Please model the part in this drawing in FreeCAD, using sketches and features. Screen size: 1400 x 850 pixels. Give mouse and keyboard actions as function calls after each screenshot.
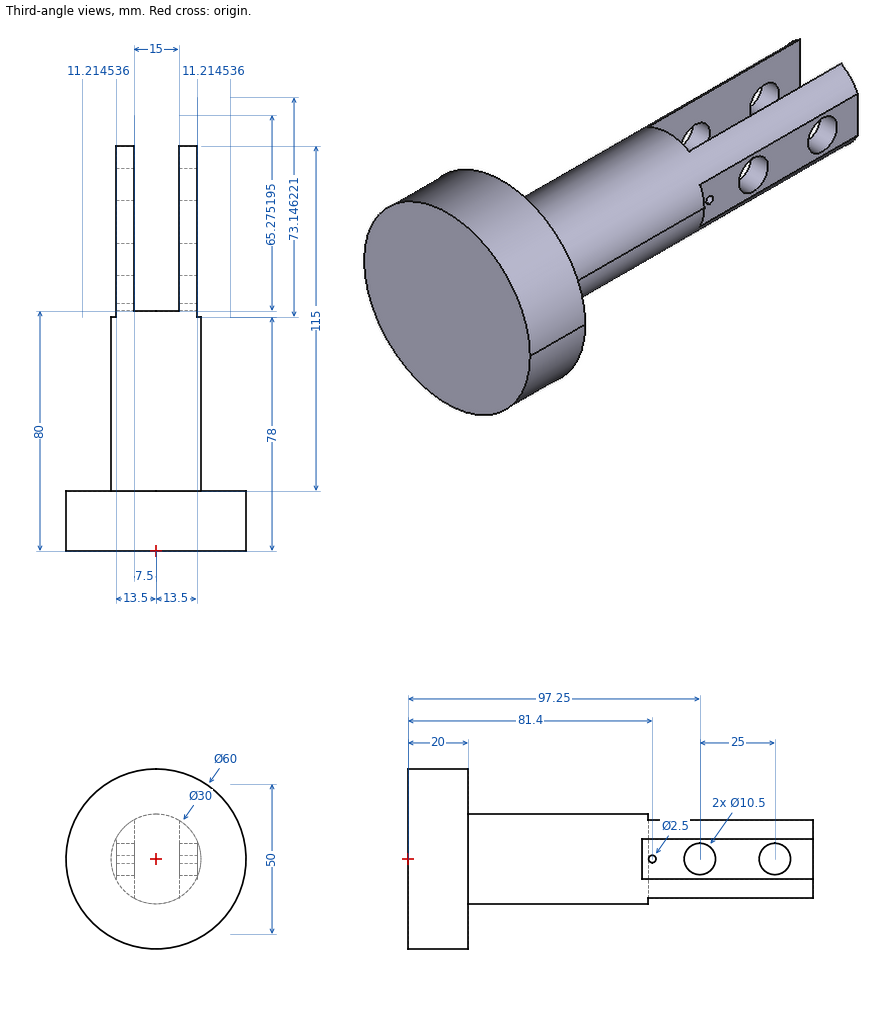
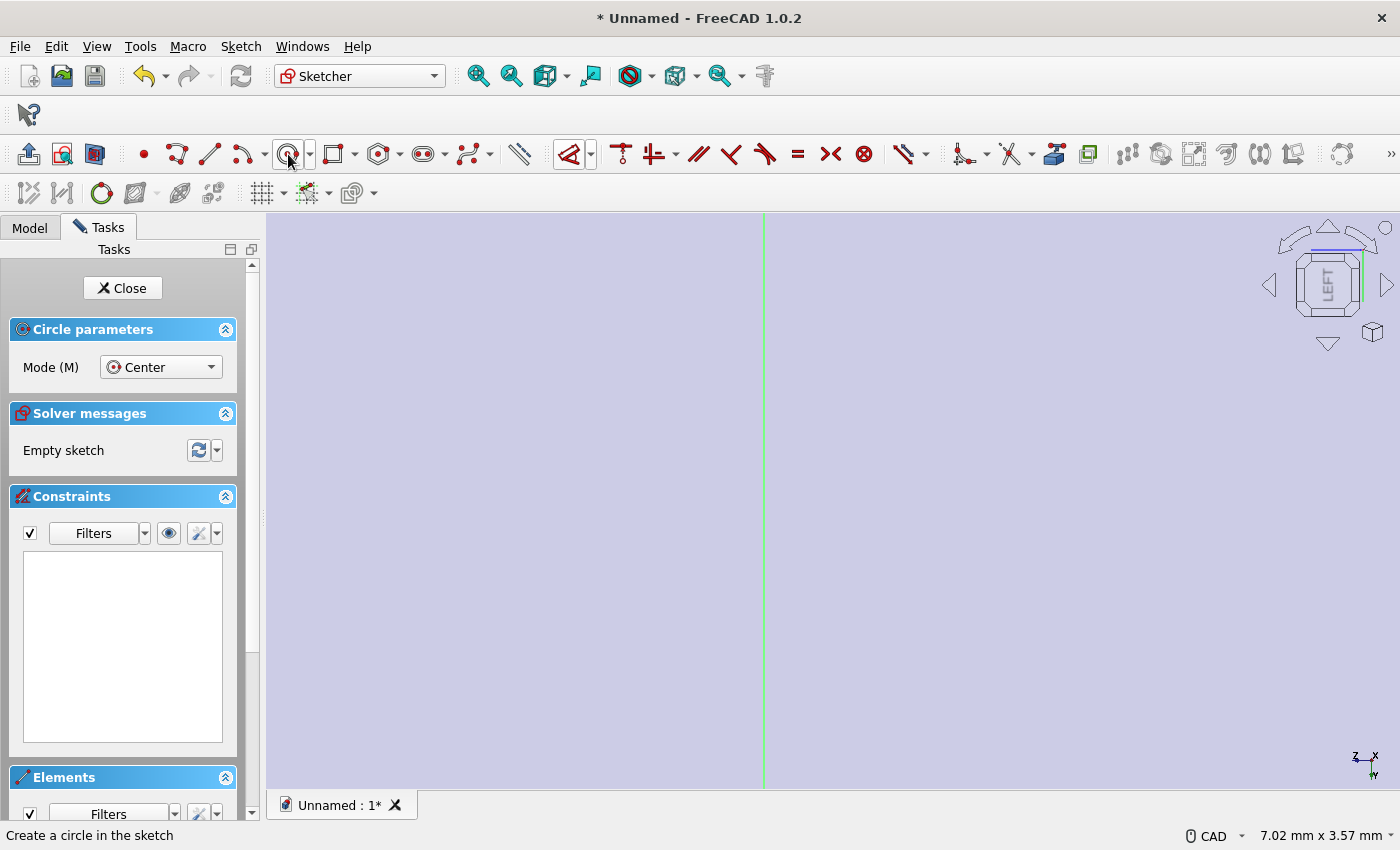
click(764, 500)
move(907, 357)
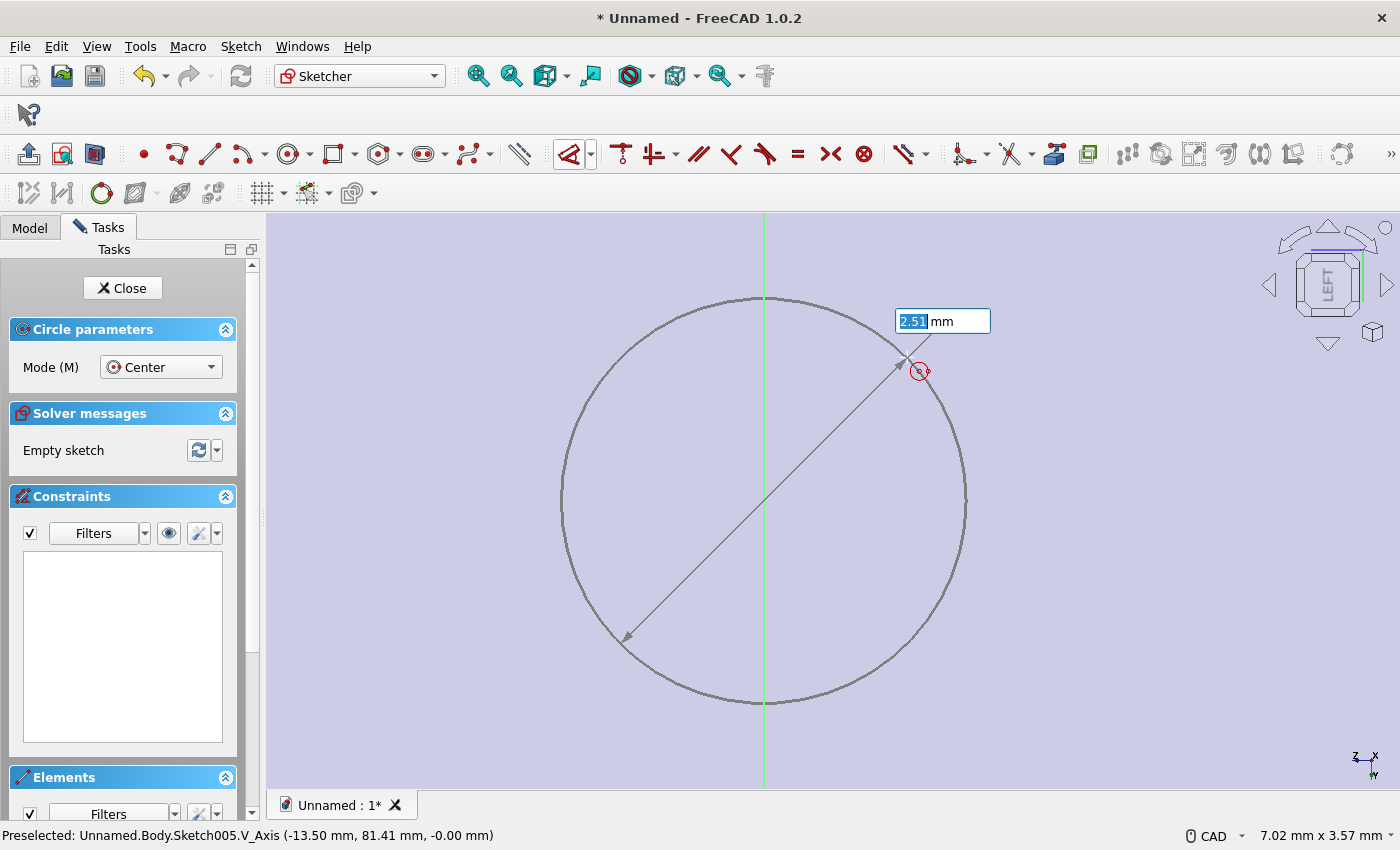
text(2.5)
key(Return)
key(Escape)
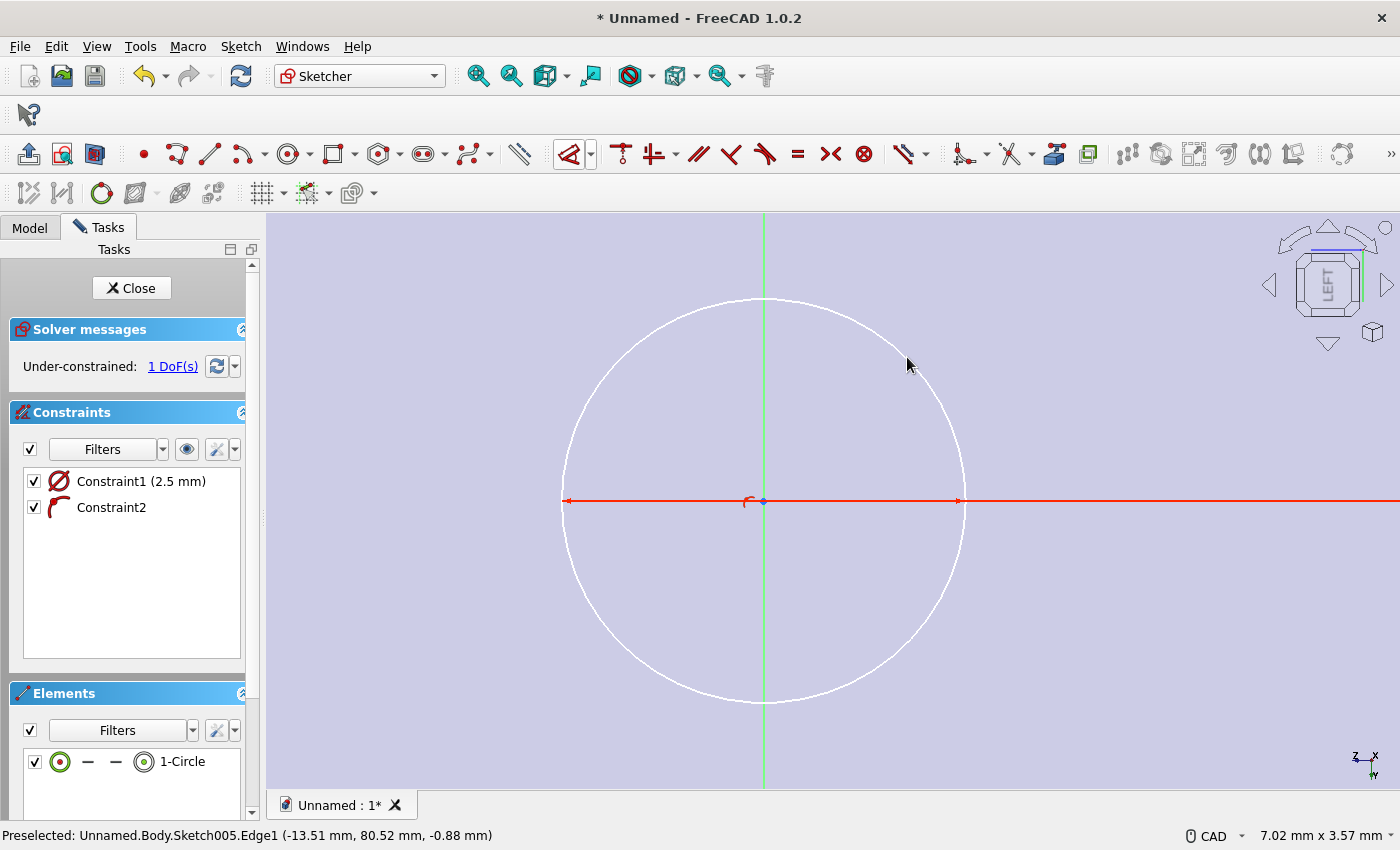
click(764, 501)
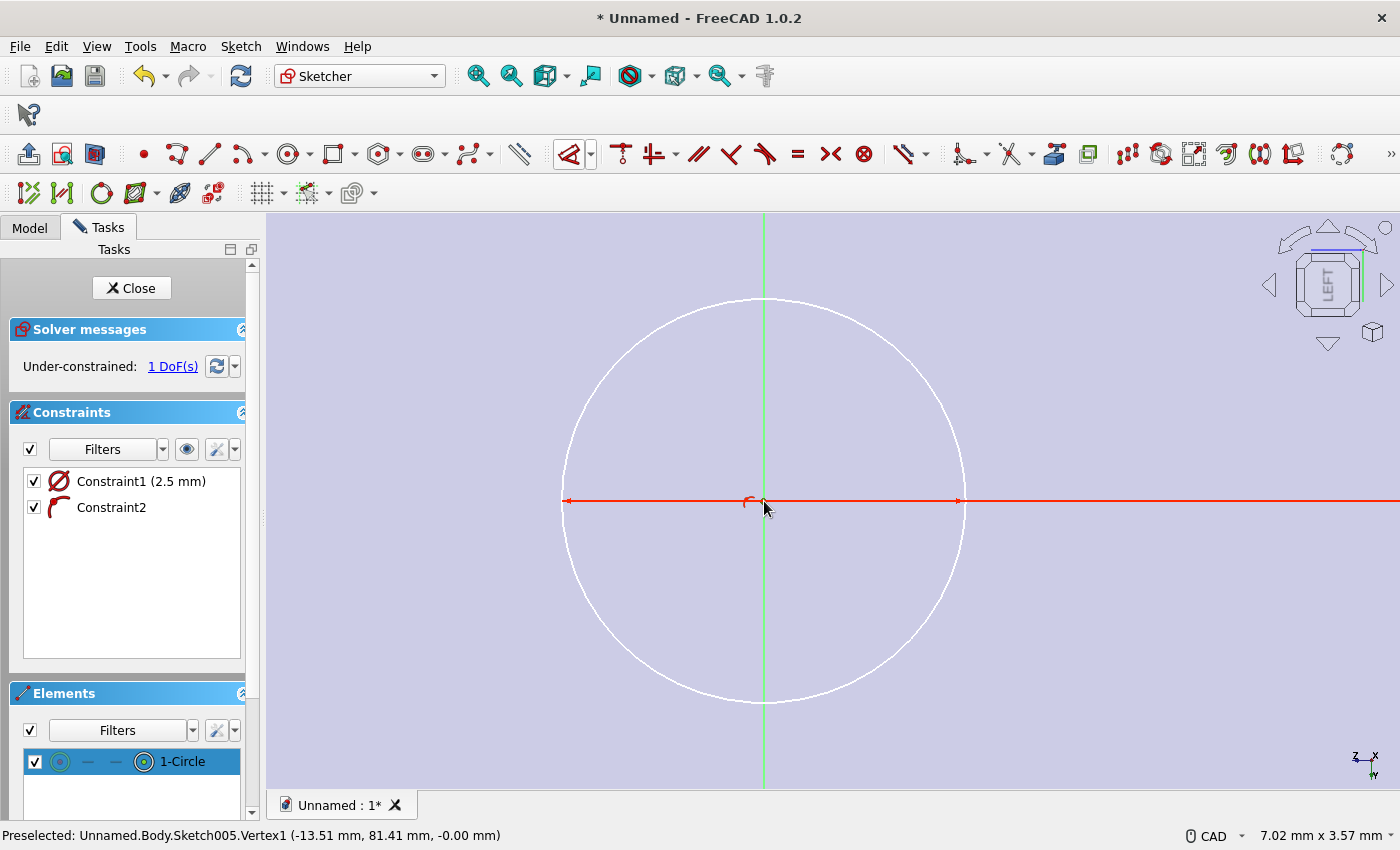
key(i)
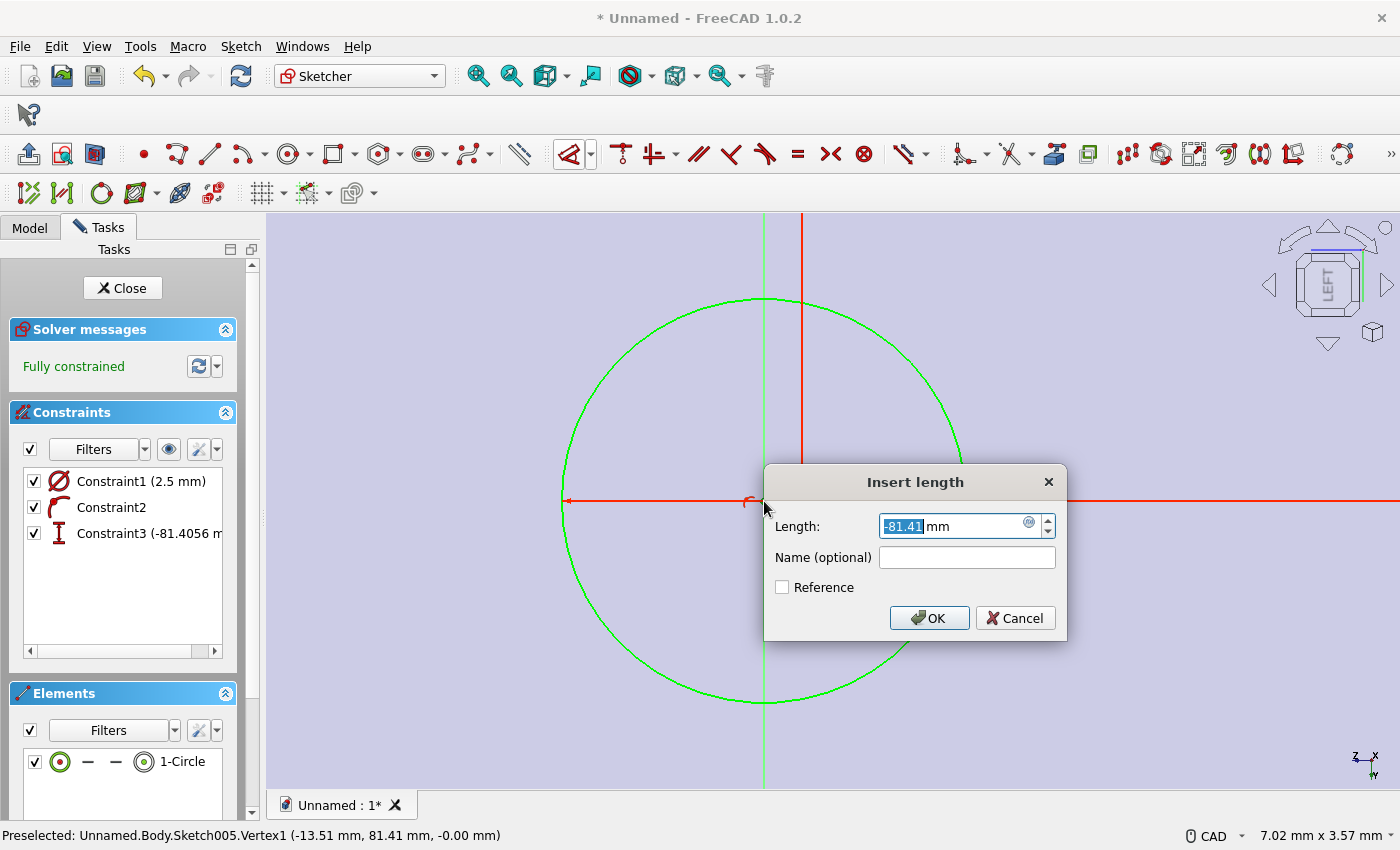
text(-81.4)
key(Return)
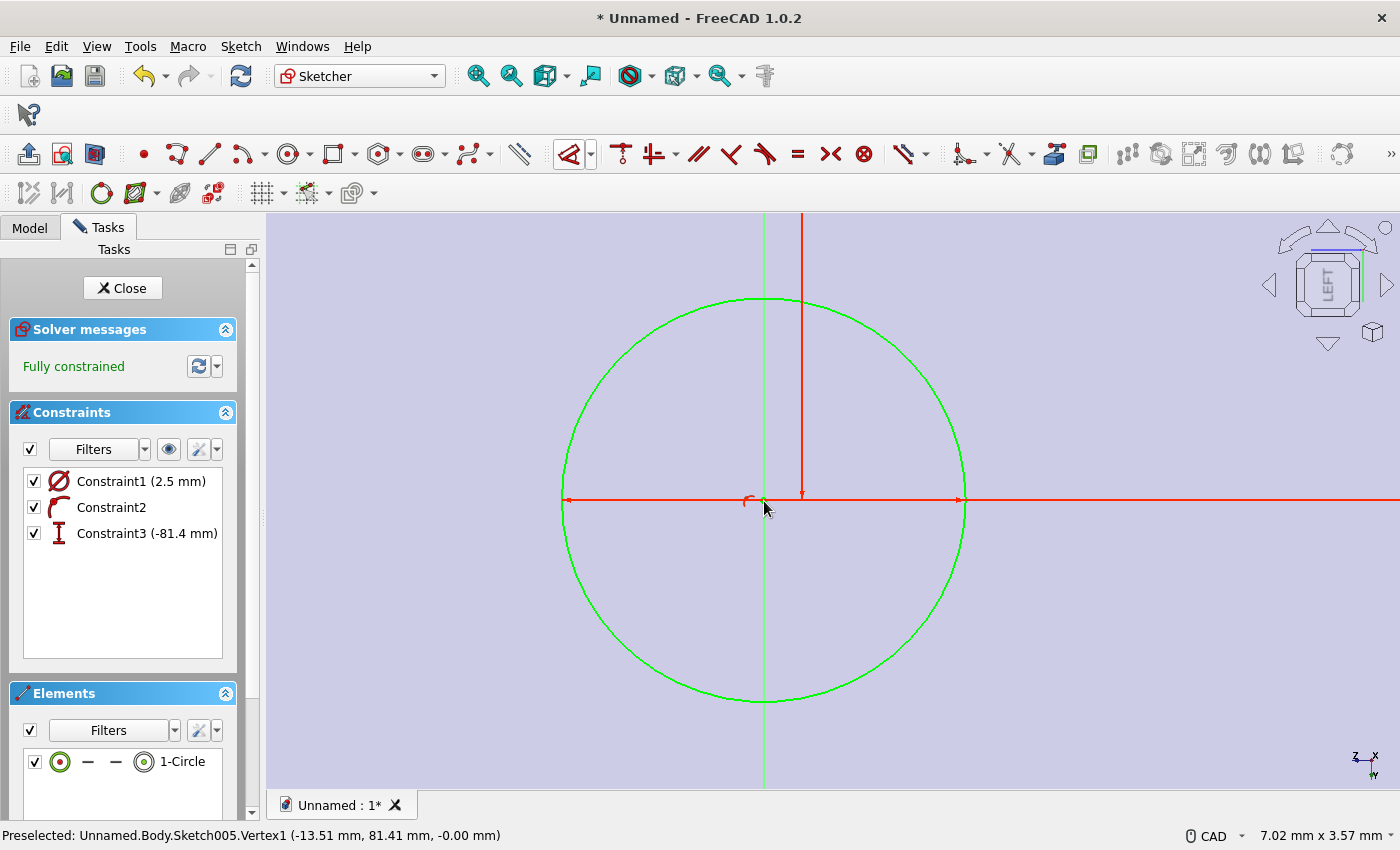
click(123, 288)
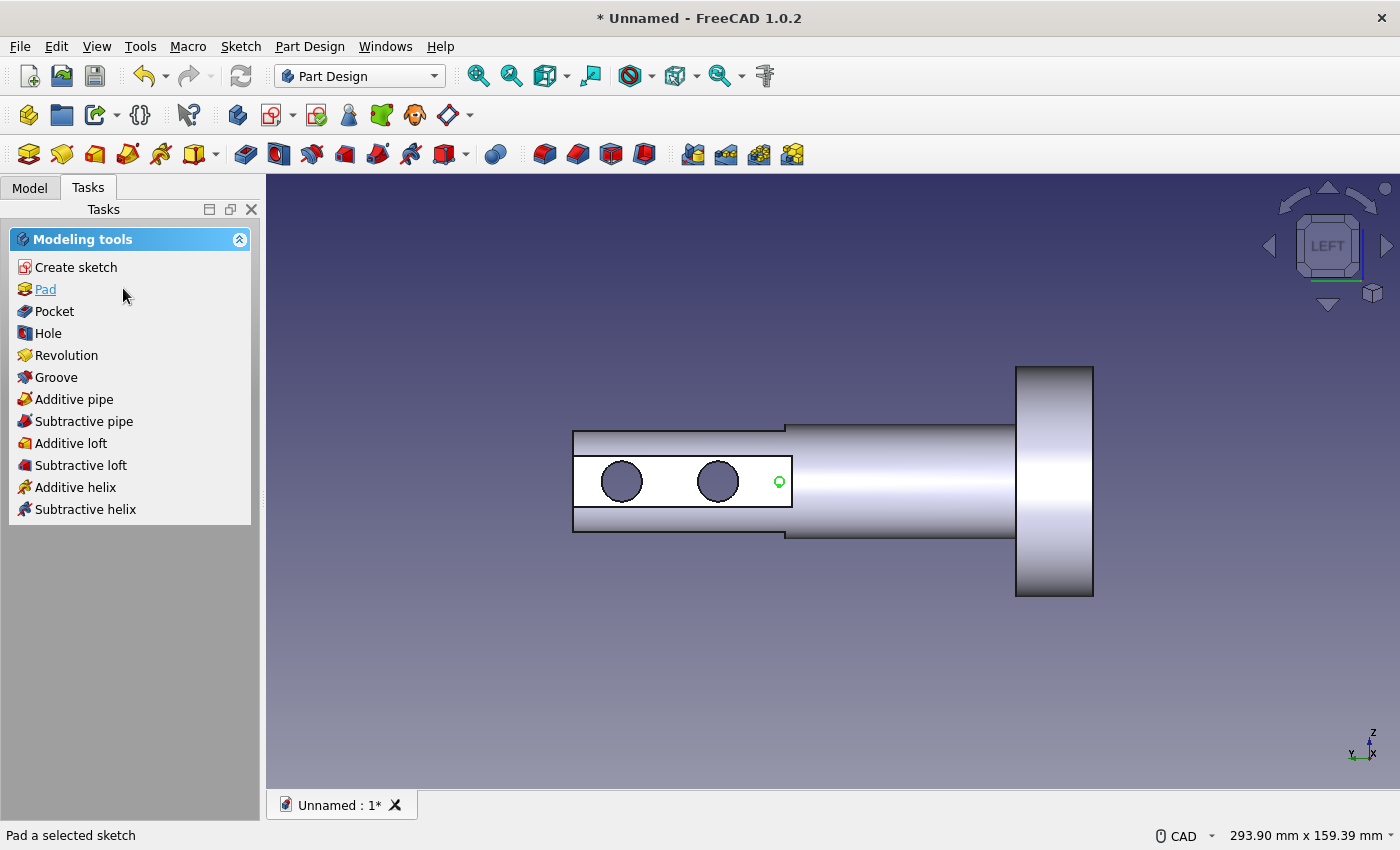
click(246, 154)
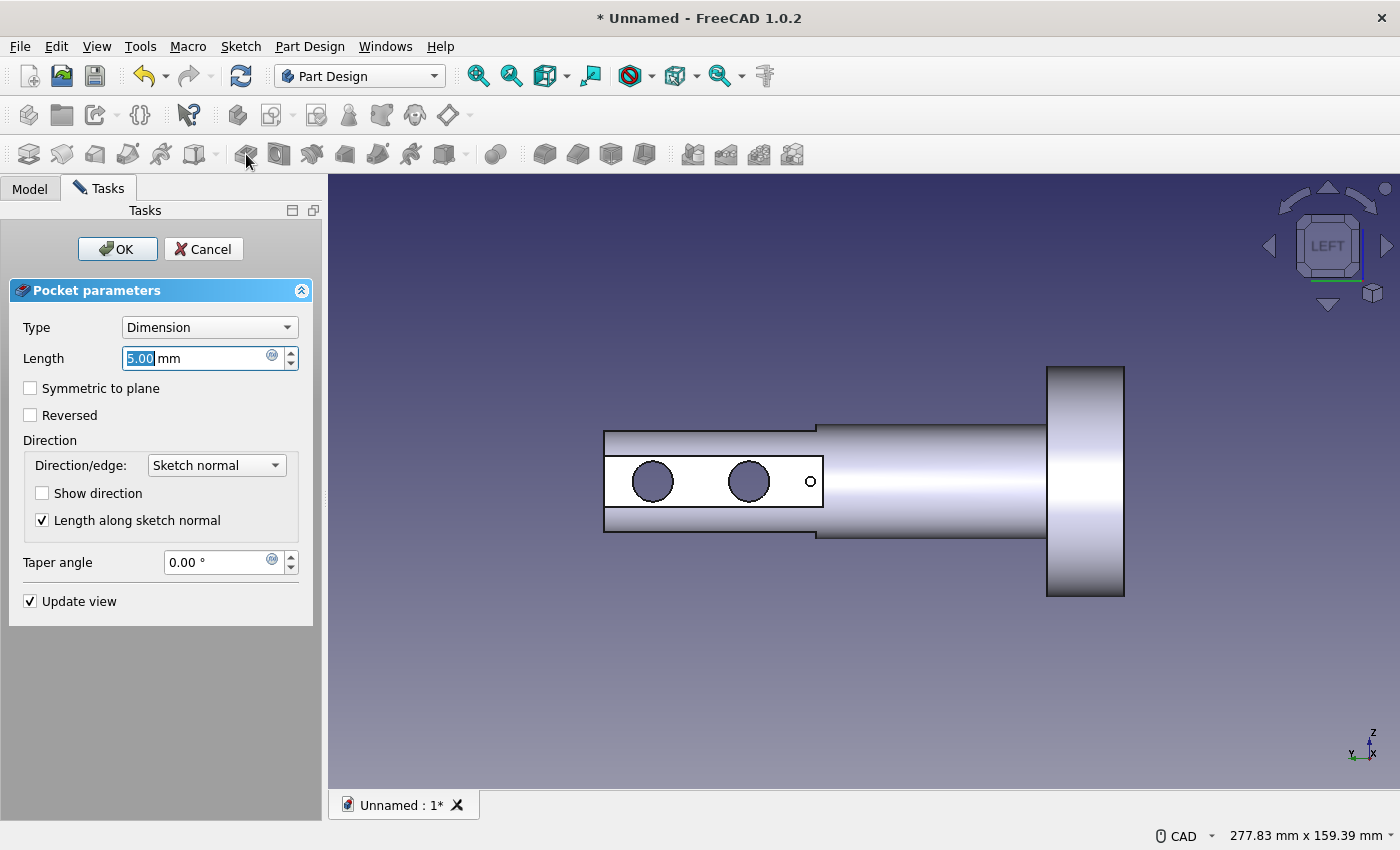
click(210, 328)